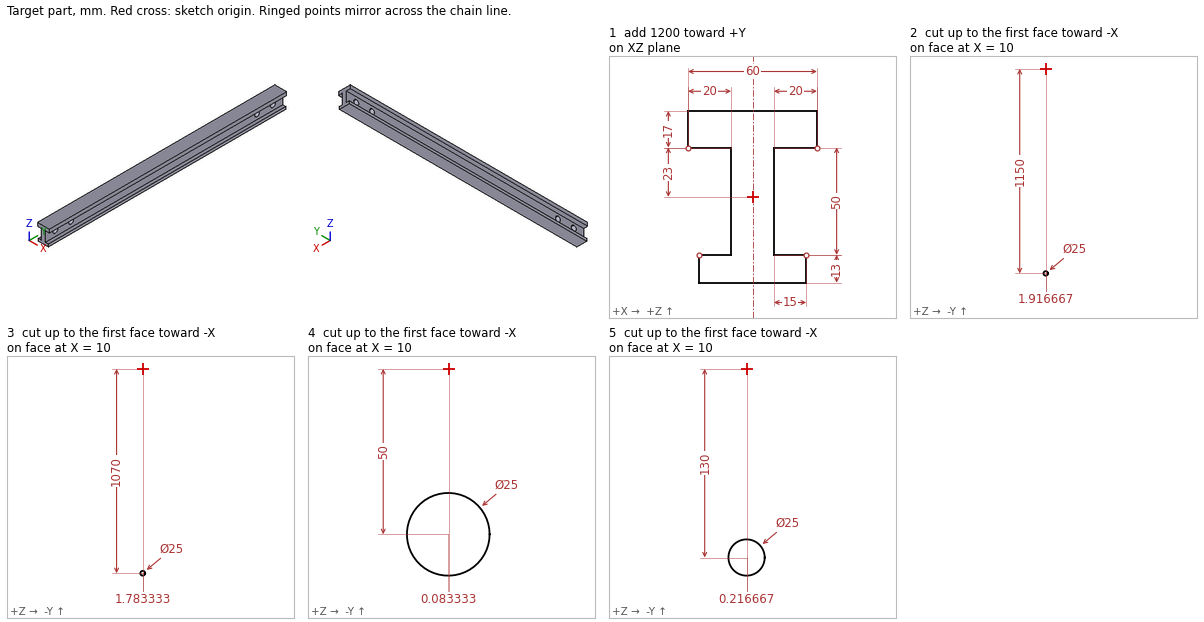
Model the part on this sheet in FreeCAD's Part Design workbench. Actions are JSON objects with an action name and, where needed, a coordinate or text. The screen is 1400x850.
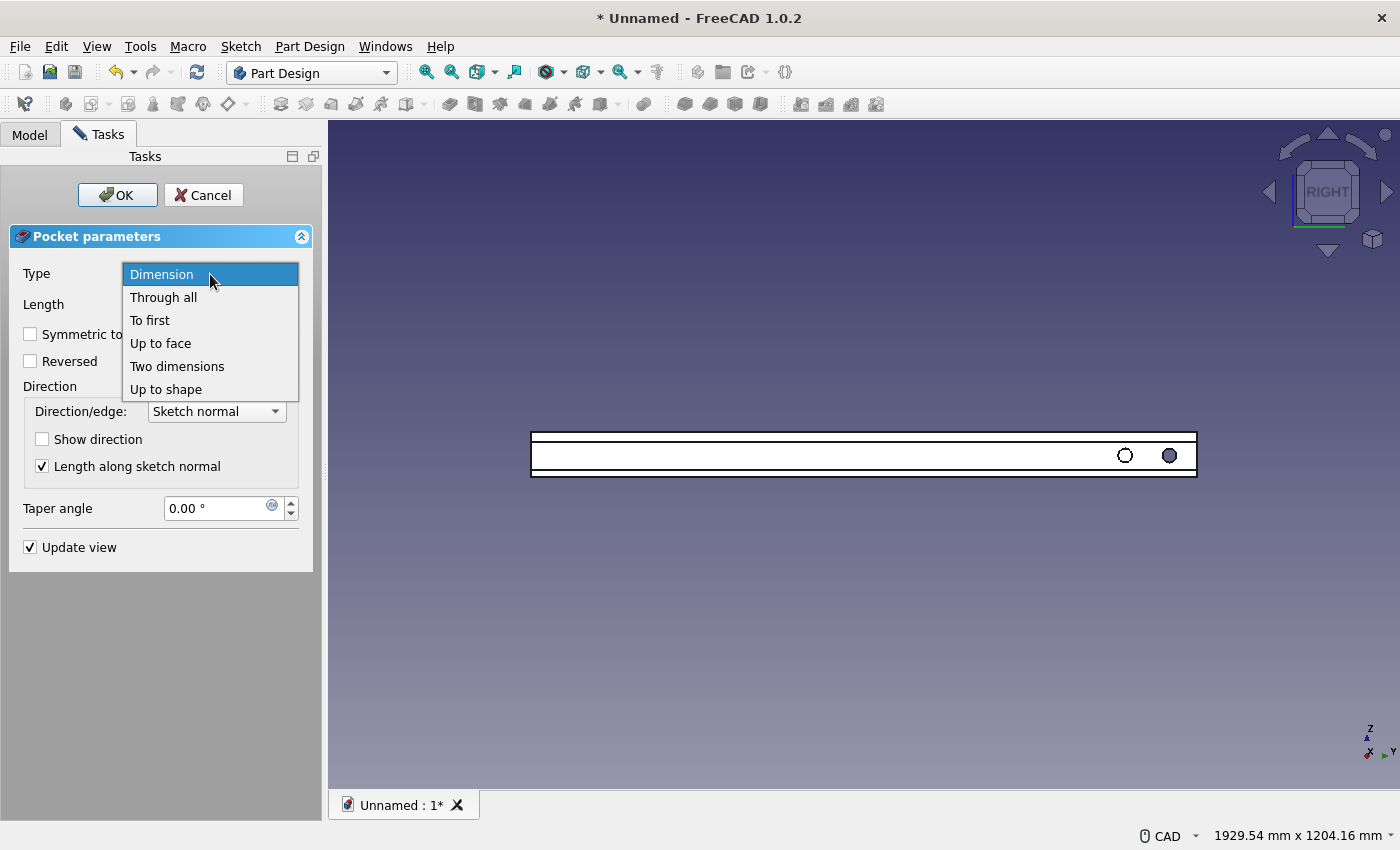
{"action": "left_click", "coordinate": [208, 320]}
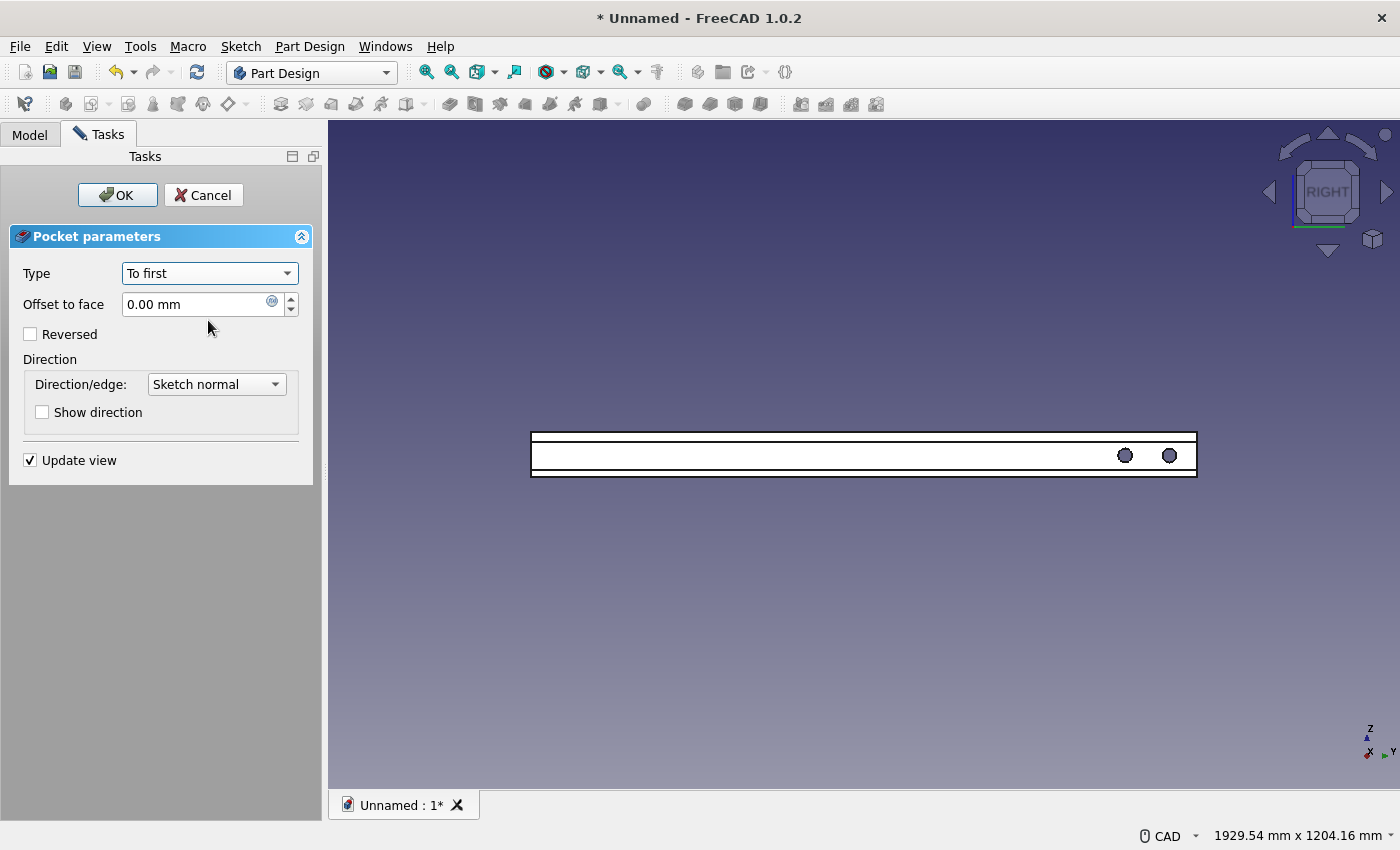
{"action": "left_click", "coordinate": [118, 195]}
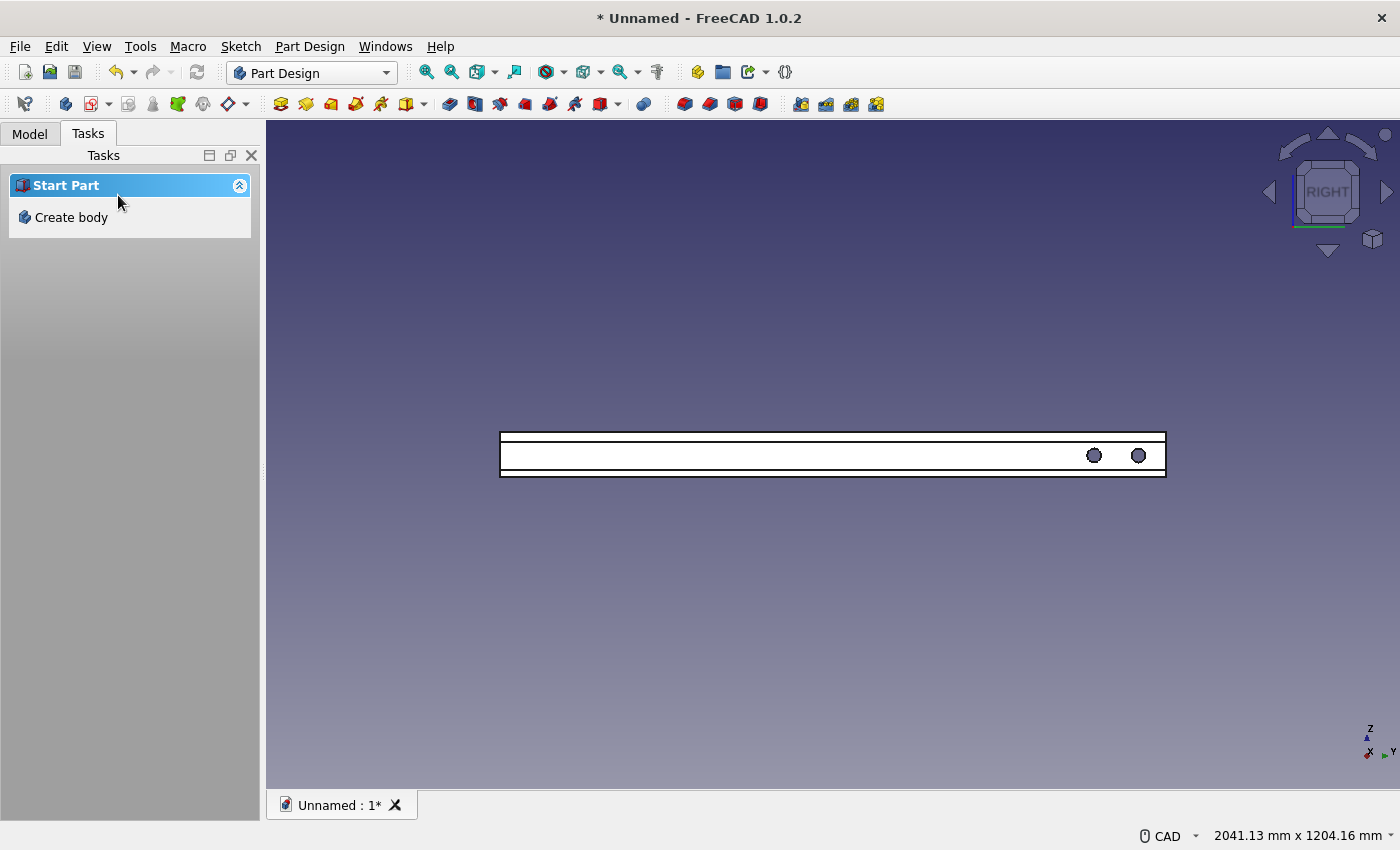
{"action": "left_click", "coordinate": [1023, 455]}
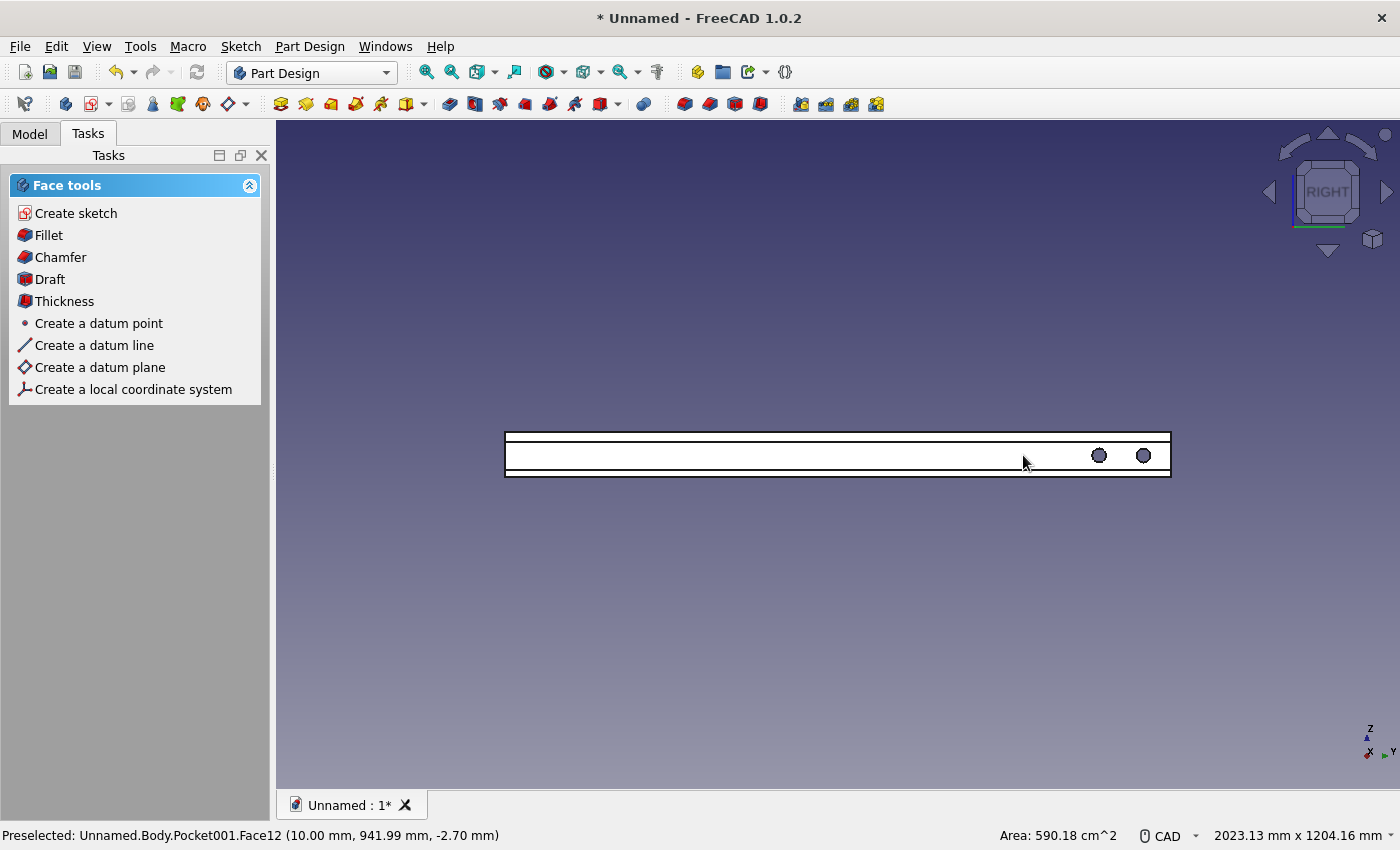
{"action": "left_click", "coordinate": [90, 104]}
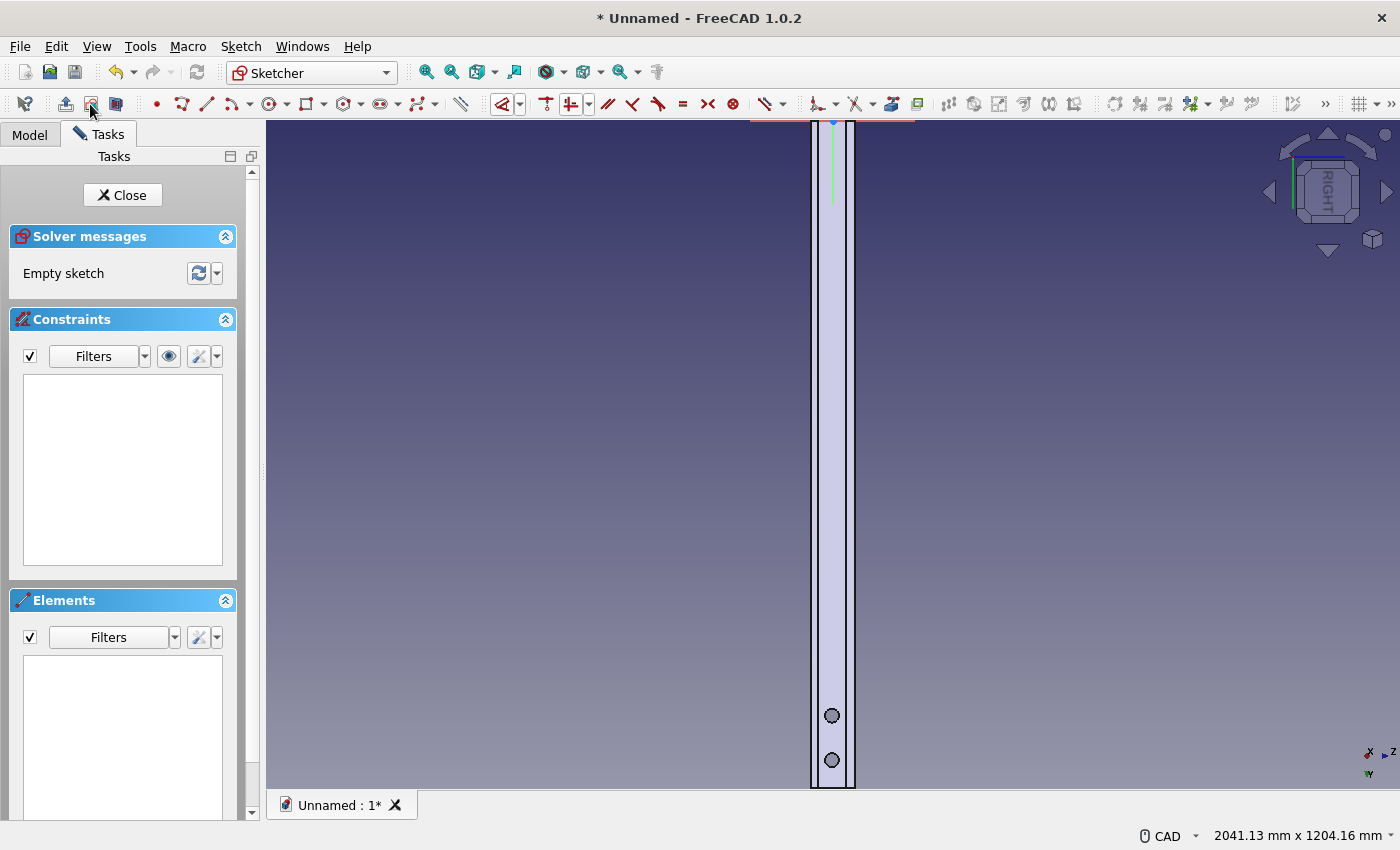
{"action": "left_click", "coordinate": [116, 104]}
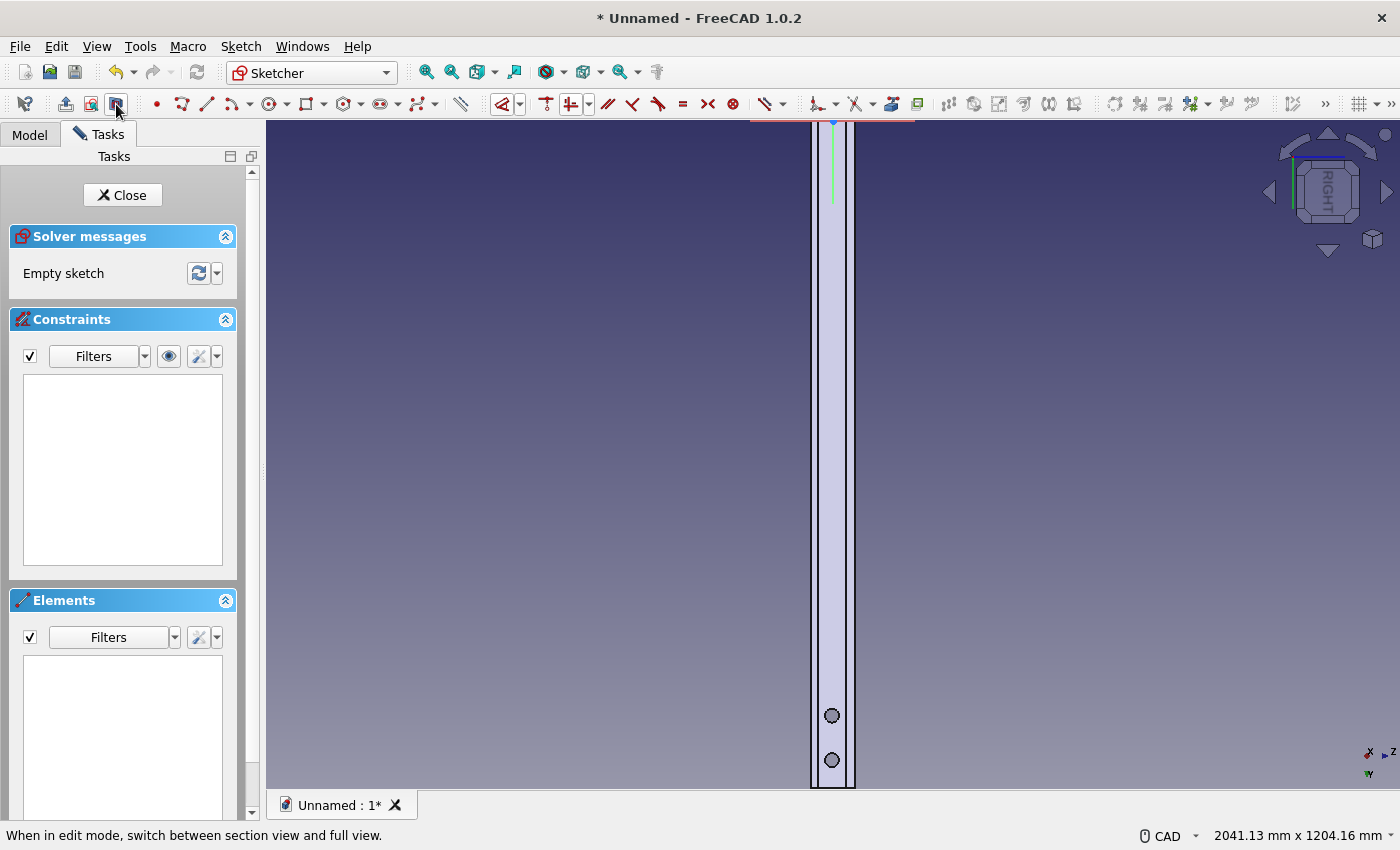
{"action": "scroll", "coordinate": [764, 454], "scroll_direction": "down", "scroll_amount": 5}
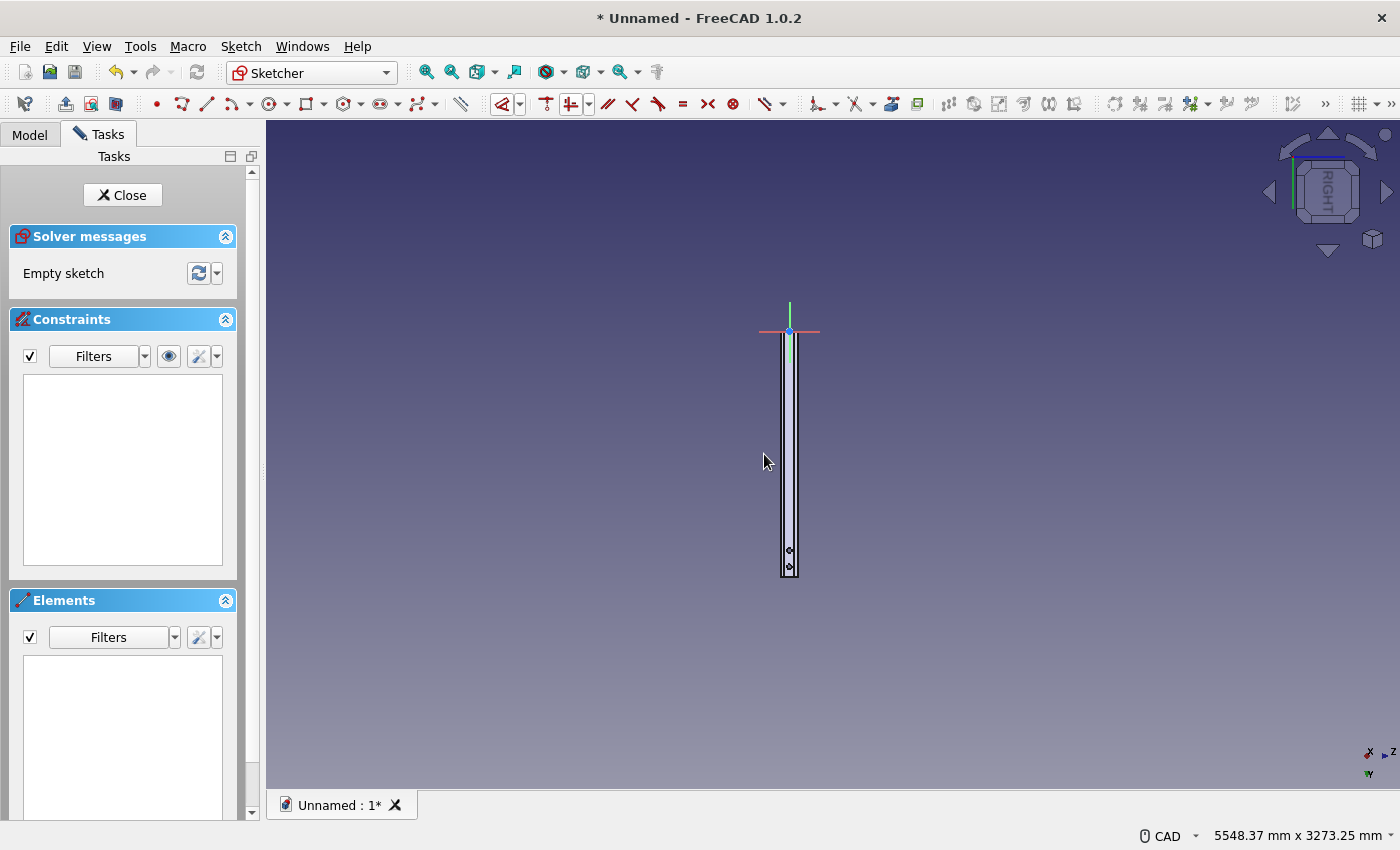
{"action": "scroll", "coordinate": [791, 336], "scroll_direction": "up", "scroll_amount": 15}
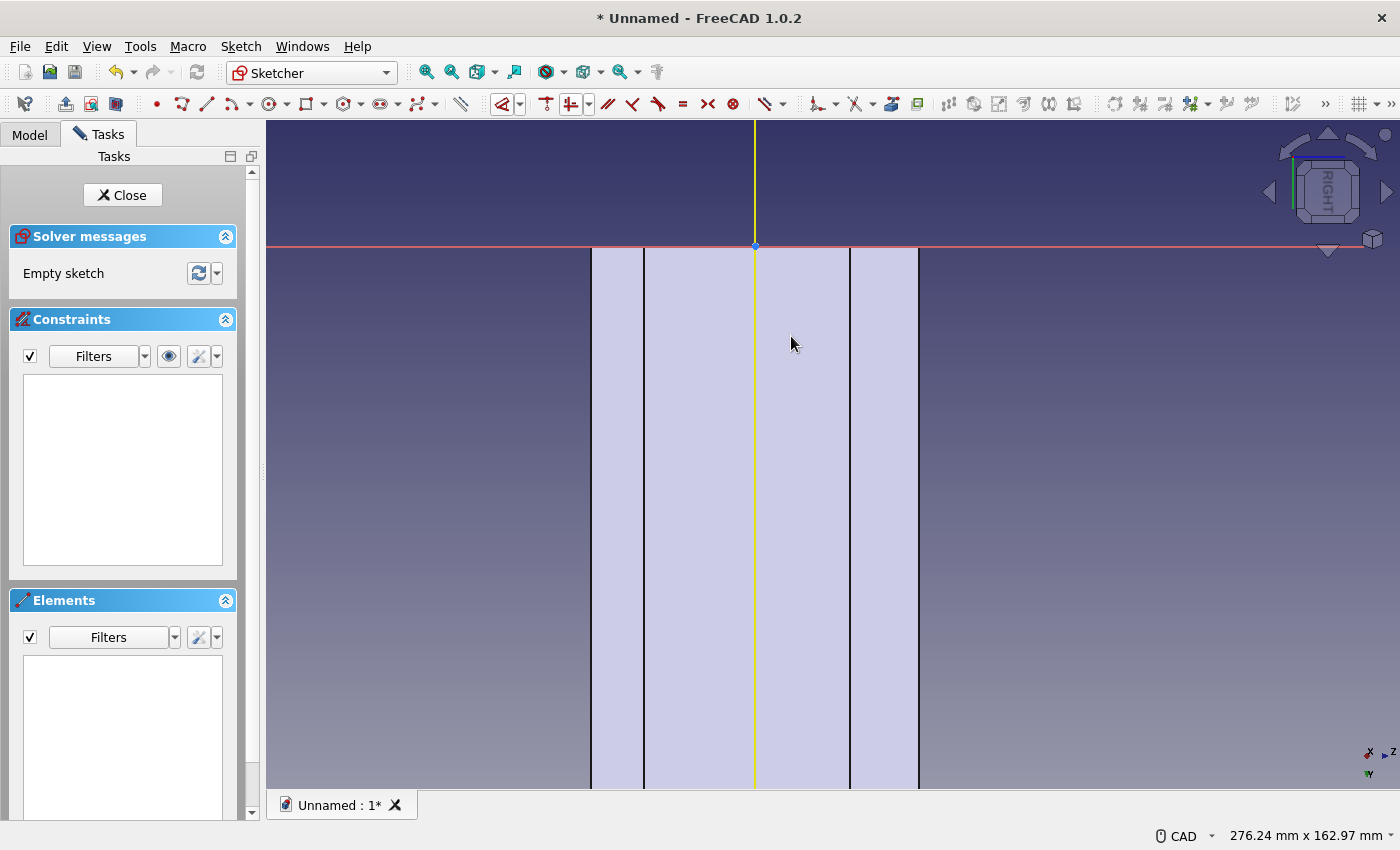
{"action": "scroll", "coordinate": [752, 451], "scroll_direction": "up", "scroll_amount": 7}